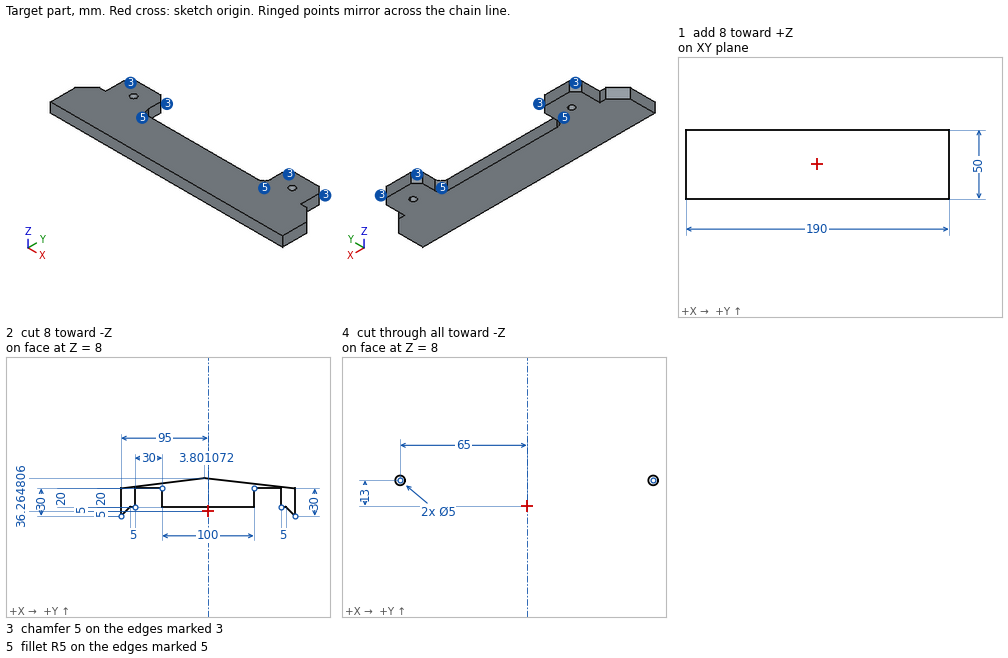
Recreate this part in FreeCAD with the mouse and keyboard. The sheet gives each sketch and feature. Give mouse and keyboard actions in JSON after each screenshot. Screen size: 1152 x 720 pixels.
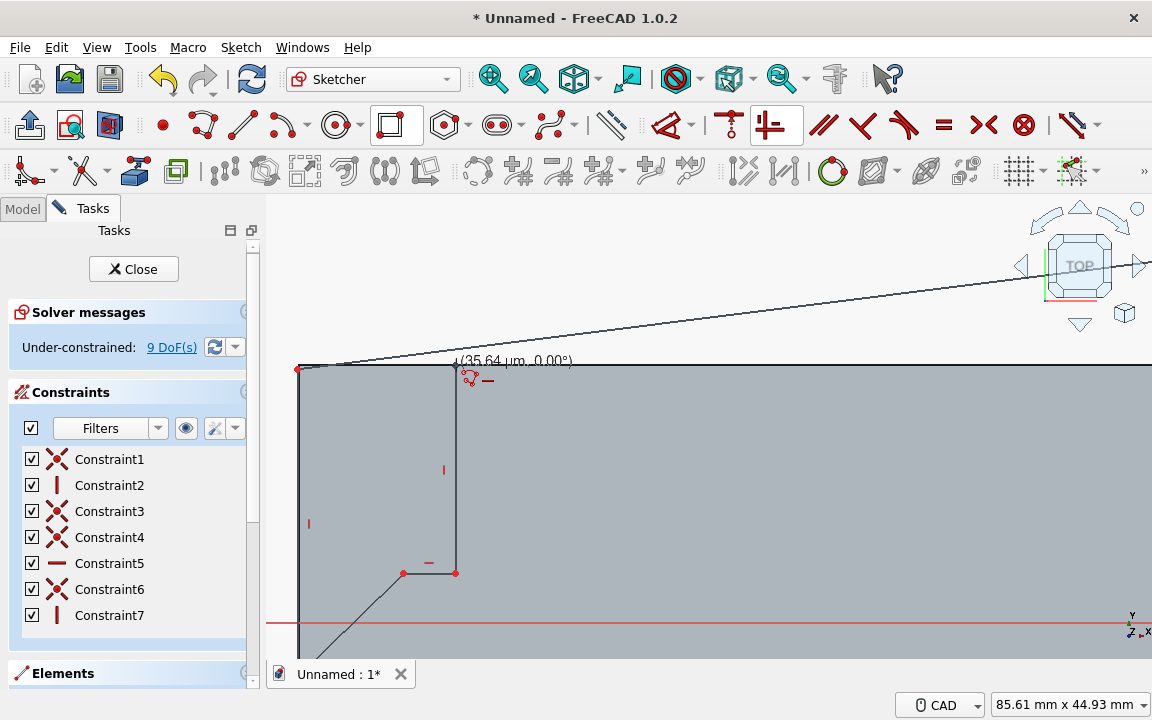
{"action": "scroll", "coordinate": [430, 415], "scroll_direction": "down", "scroll_amount": 7}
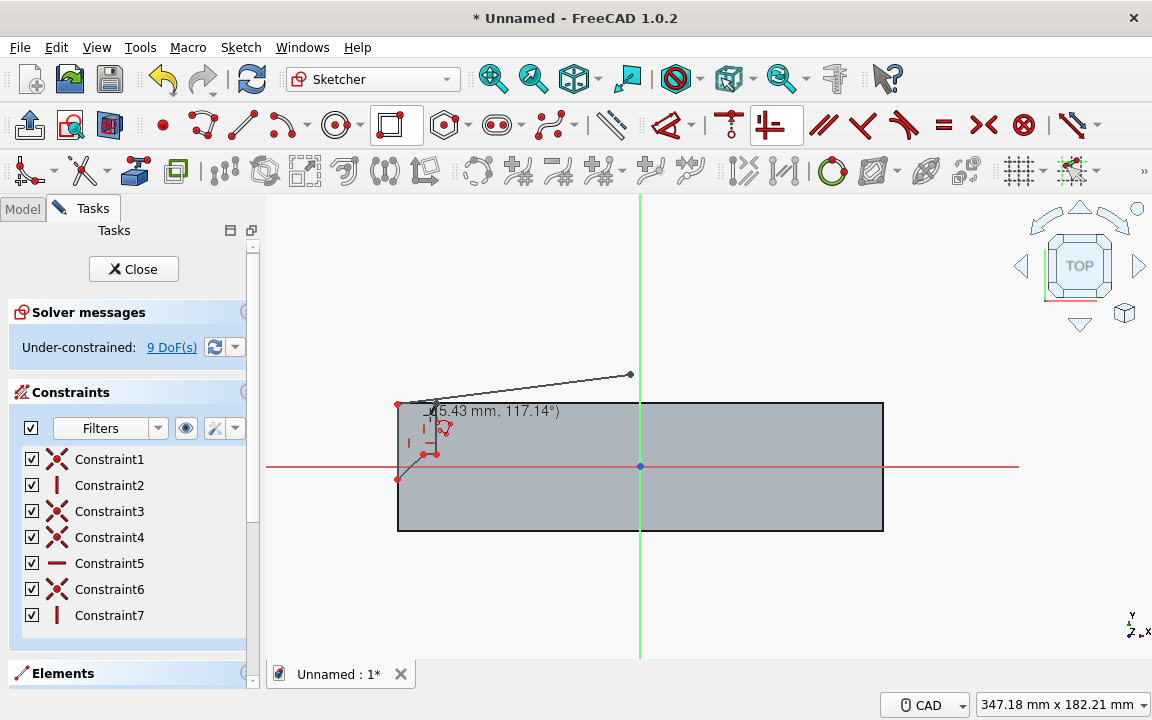
{"action": "left_click", "coordinate": [513, 403]}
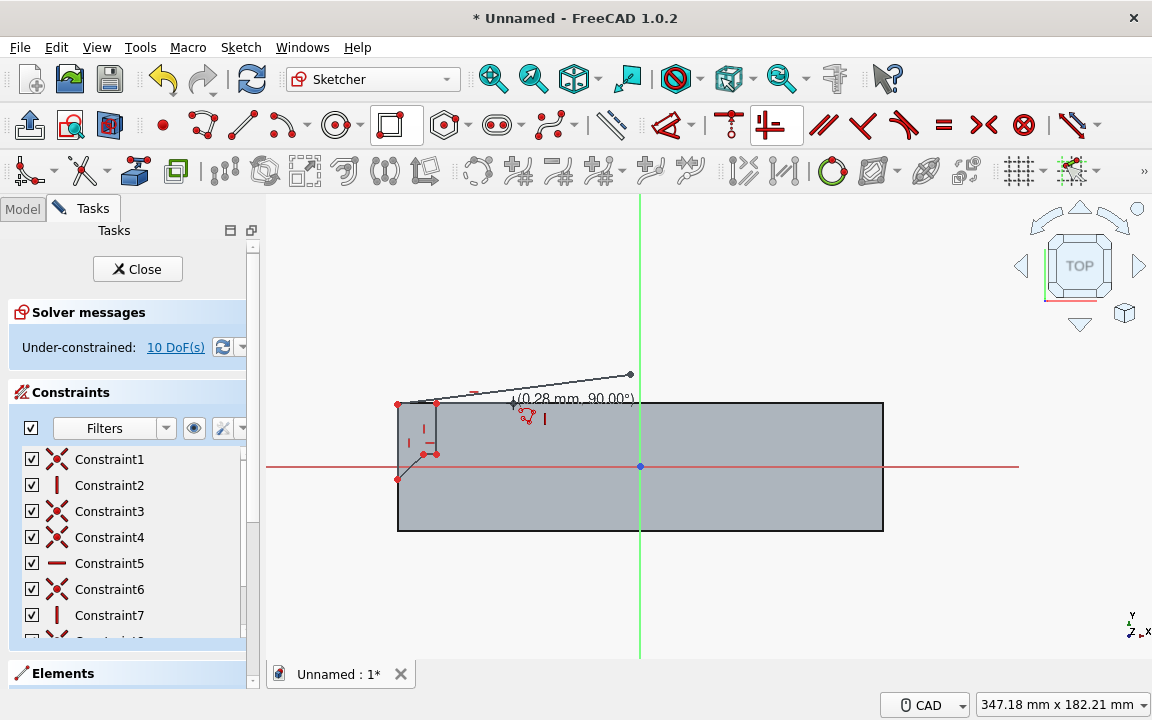
{"action": "scroll", "coordinate": [513, 454], "scroll_direction": "up", "scroll_amount": 2}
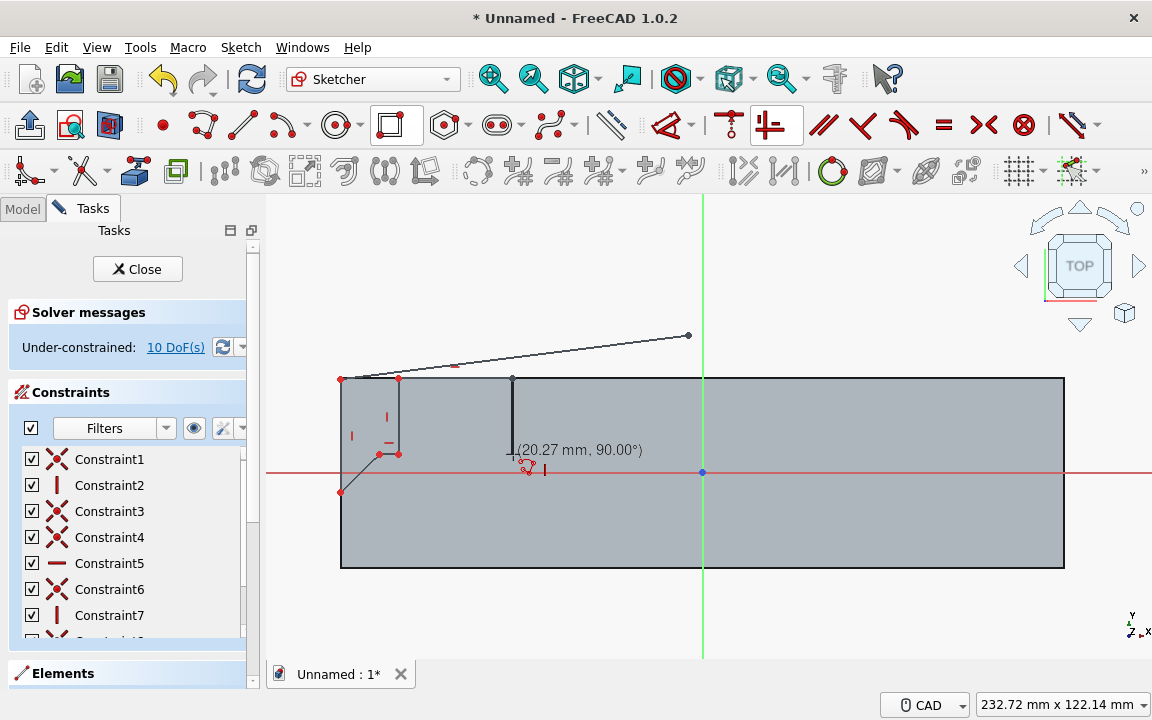
{"action": "left_click", "coordinate": [513, 454]}
{"action": "left_click", "coordinate": [893, 454]}
{"action": "left_click", "coordinate": [893, 378]}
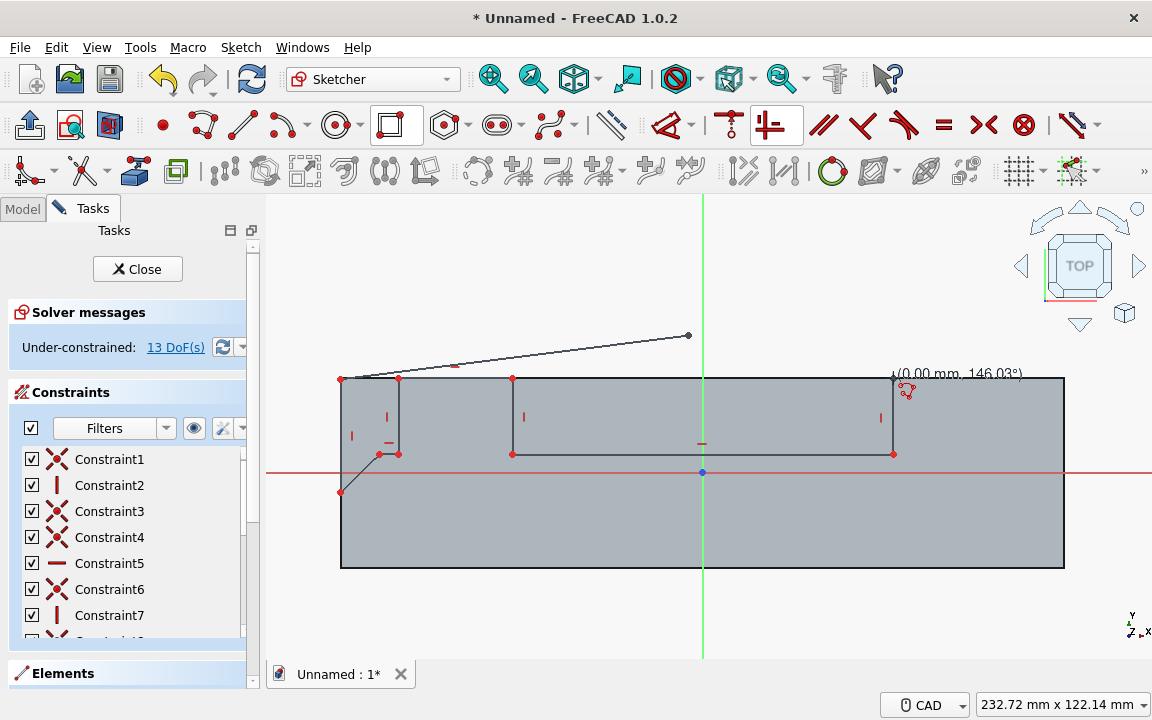
{"action": "scroll", "coordinate": [514, 454], "scroll_direction": "down", "scroll_amount": 2}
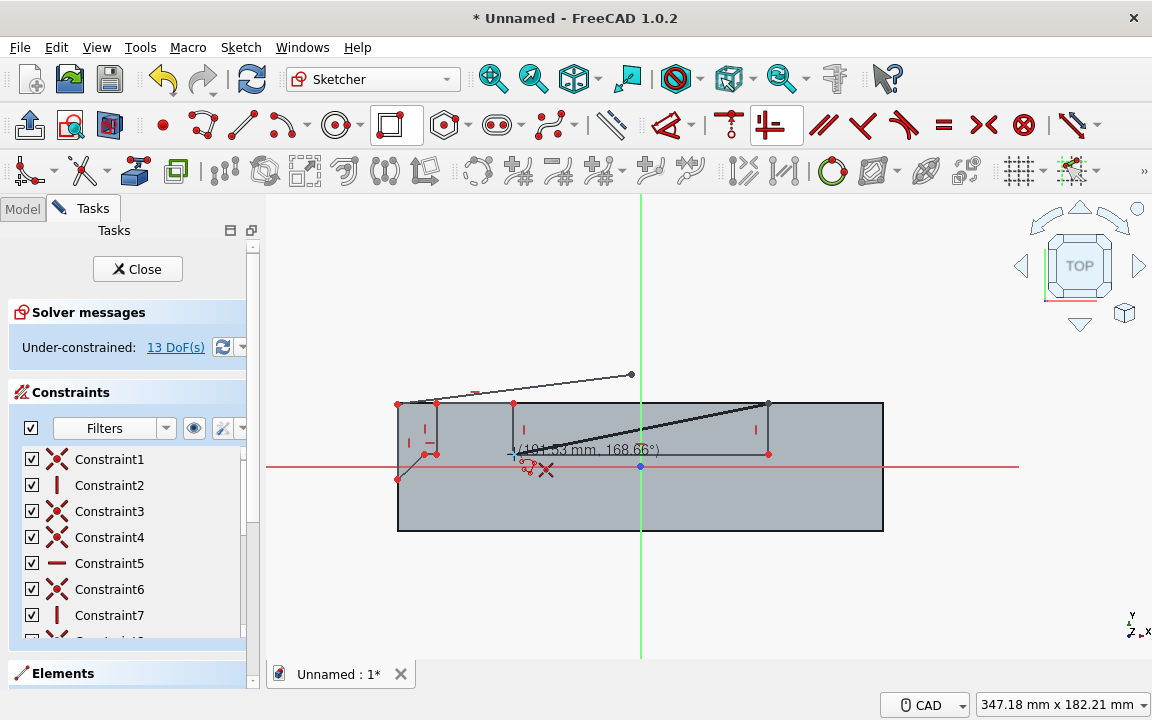
{"action": "left_click", "coordinate": [845, 403]}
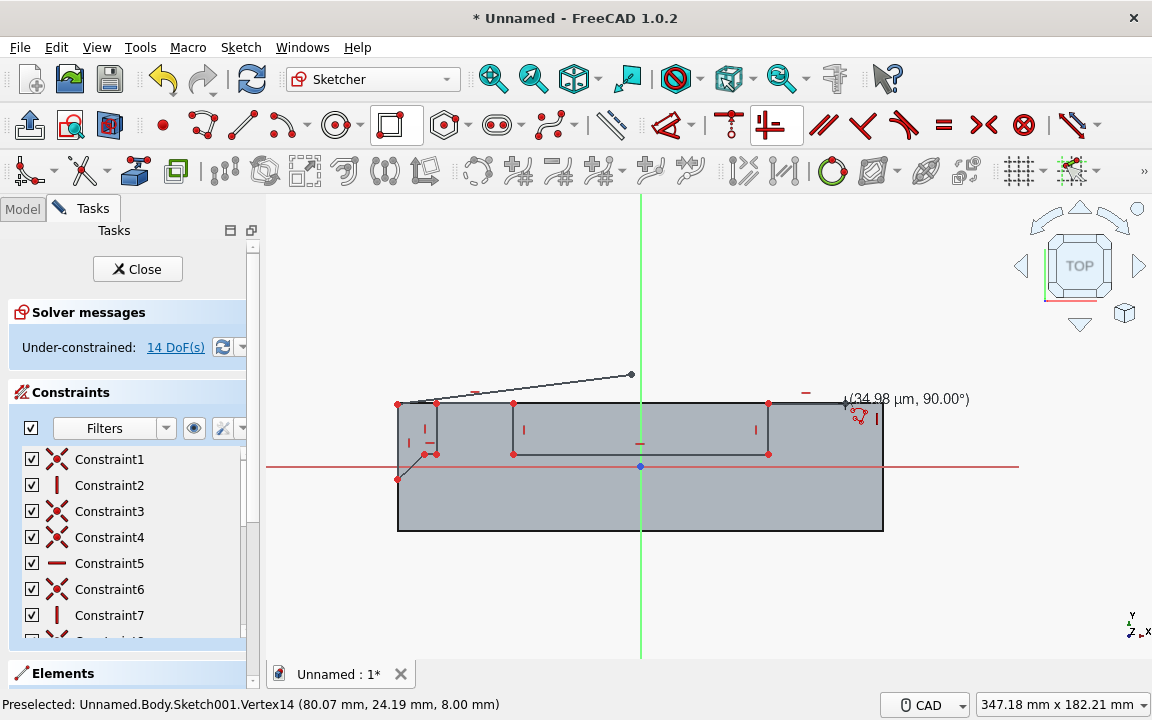
{"action": "scroll", "coordinate": [845, 454], "scroll_direction": "up", "scroll_amount": 2}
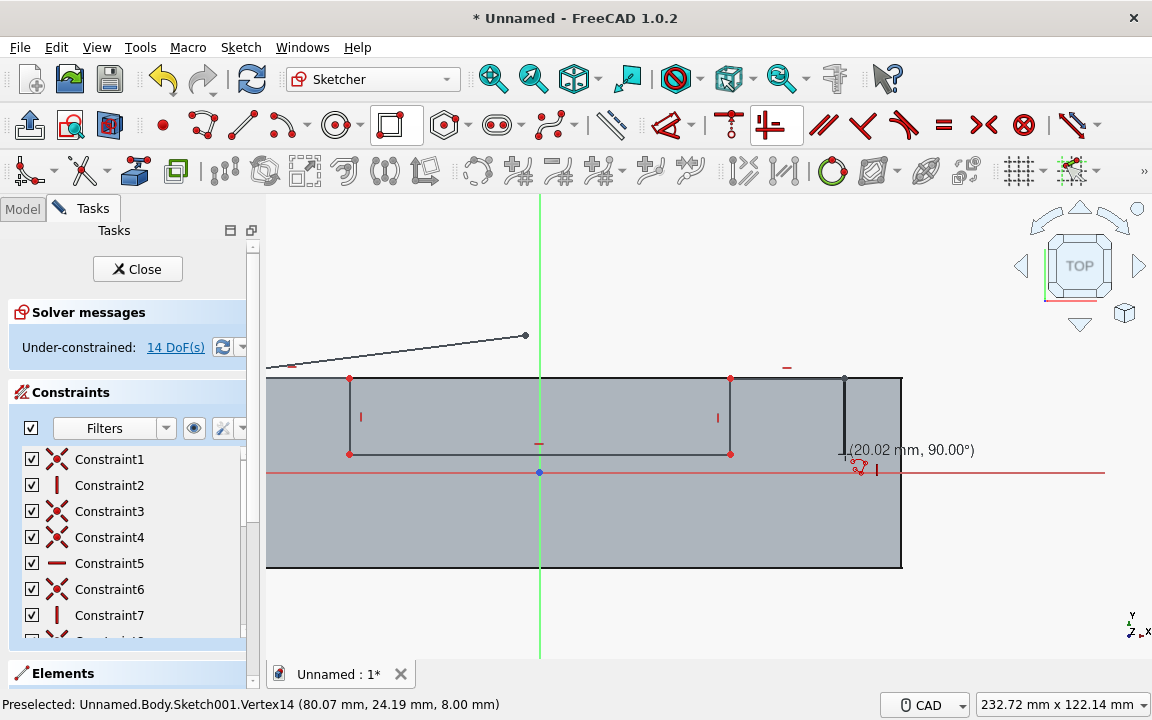
{"action": "left_click", "coordinate": [845, 454]}
{"action": "left_click", "coordinate": [863, 454]}
{"action": "left_click", "coordinate": [901, 492]}
{"action": "left_click", "coordinate": [901, 378]}
{"action": "left_click", "coordinate": [526, 336]}
{"action": "key", "text": "Escape"}
{"action": "key", "text": "Escape"}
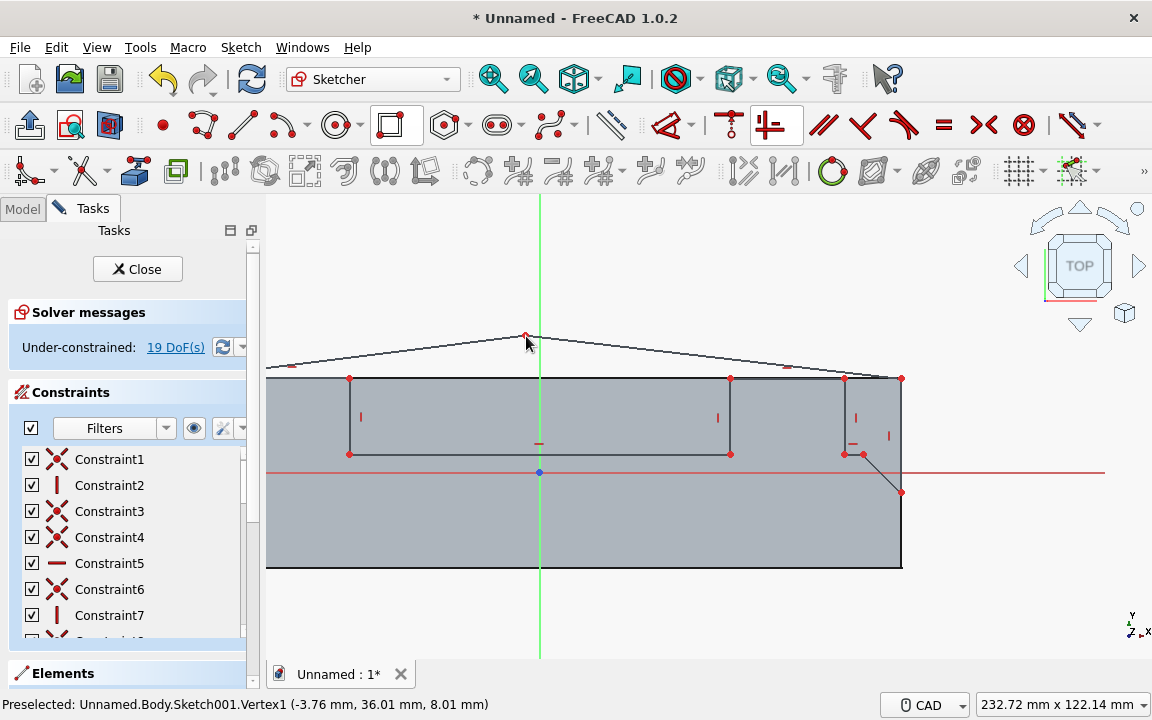
{"action": "left_click", "coordinate": [350, 378]}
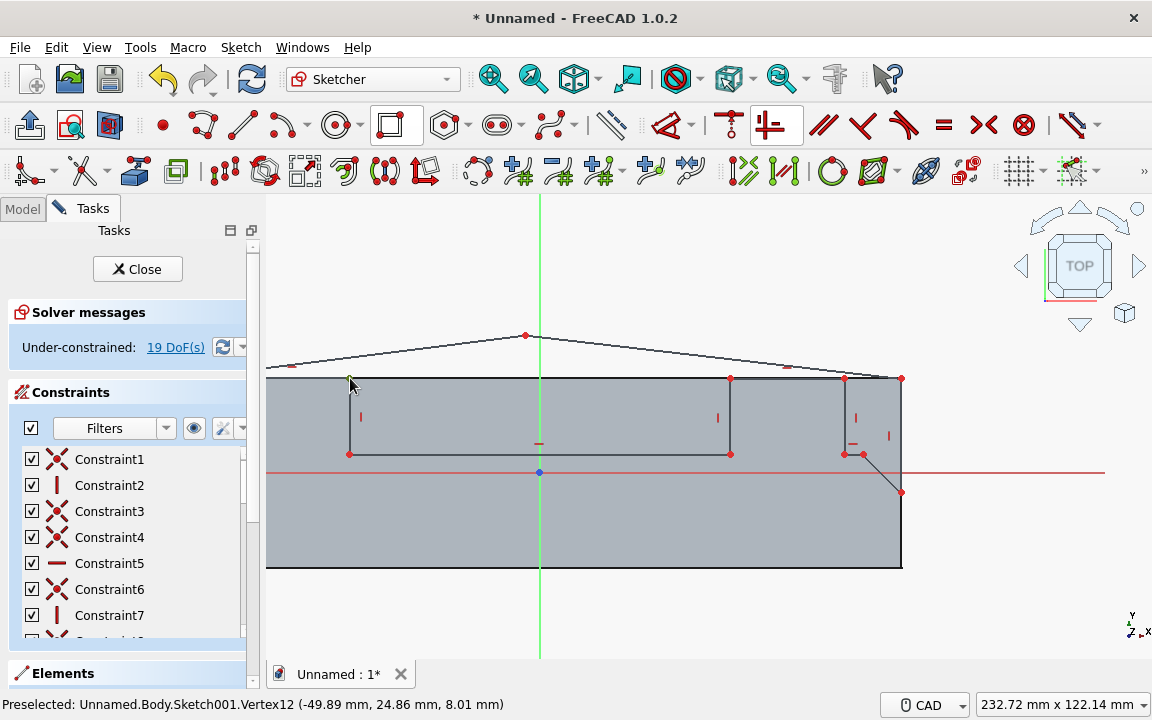
{"action": "left_click", "coordinate": [730, 379]}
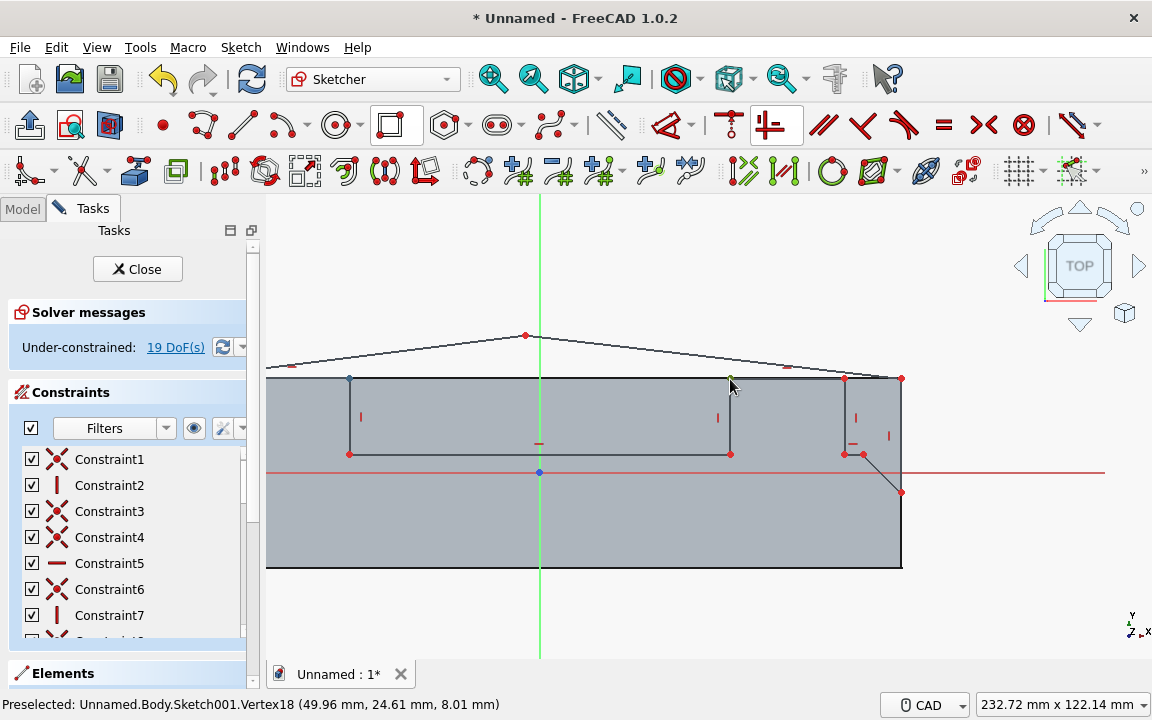
{"action": "left_click", "coordinate": [540, 602]}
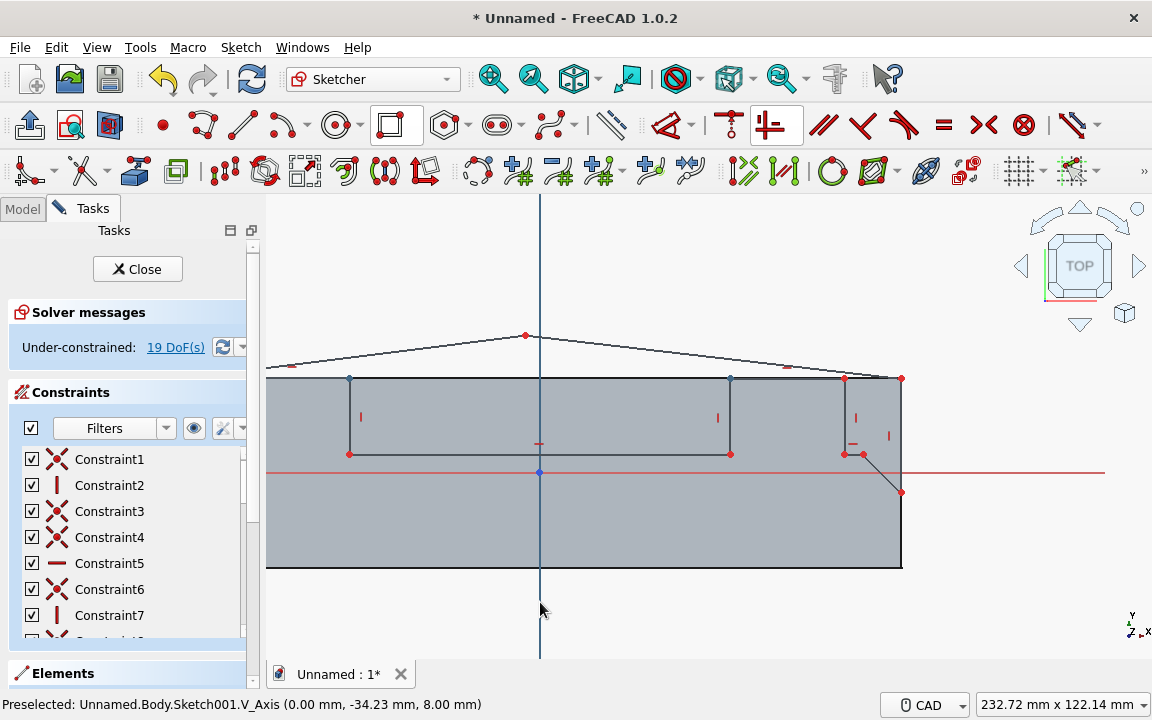
{"action": "left_click", "coordinate": [984, 126]}